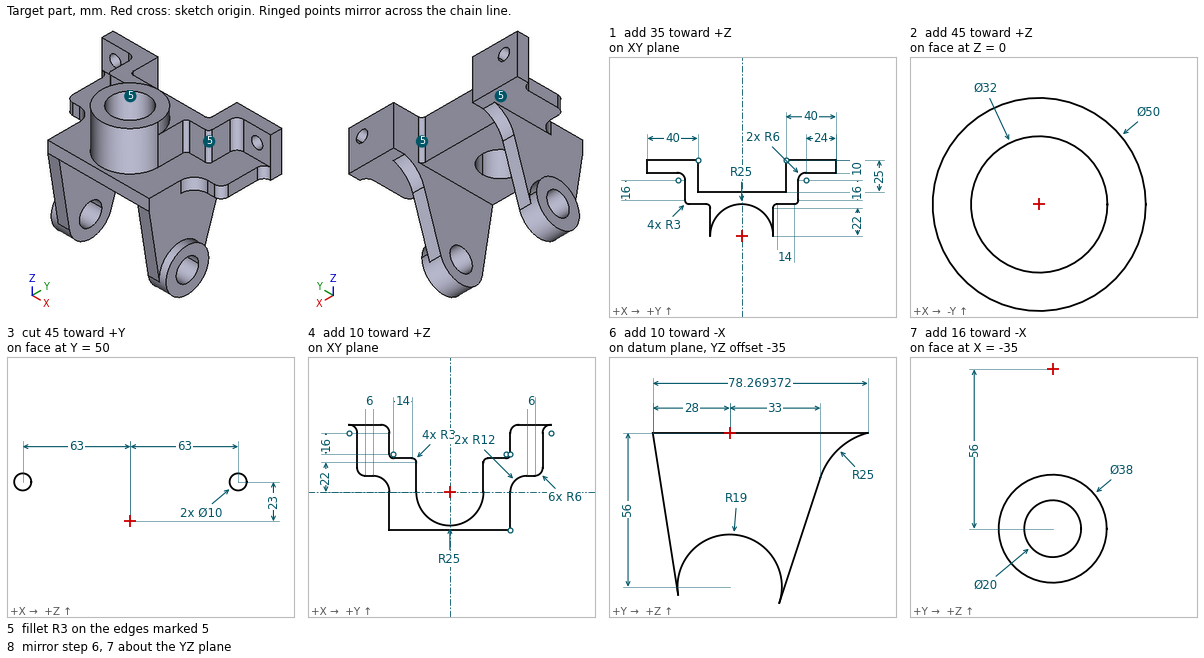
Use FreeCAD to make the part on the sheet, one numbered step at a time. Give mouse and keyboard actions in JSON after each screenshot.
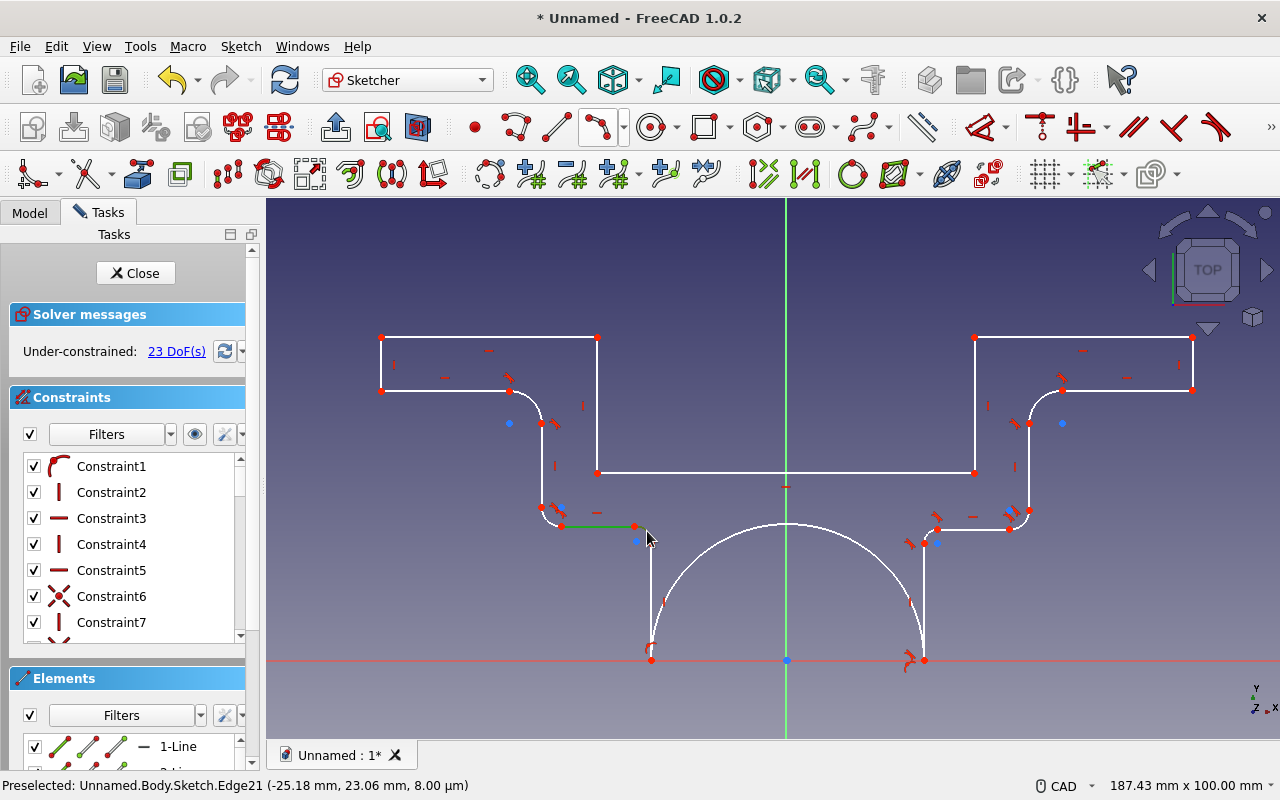
{"action": "left_click", "coordinate": [1216, 128]}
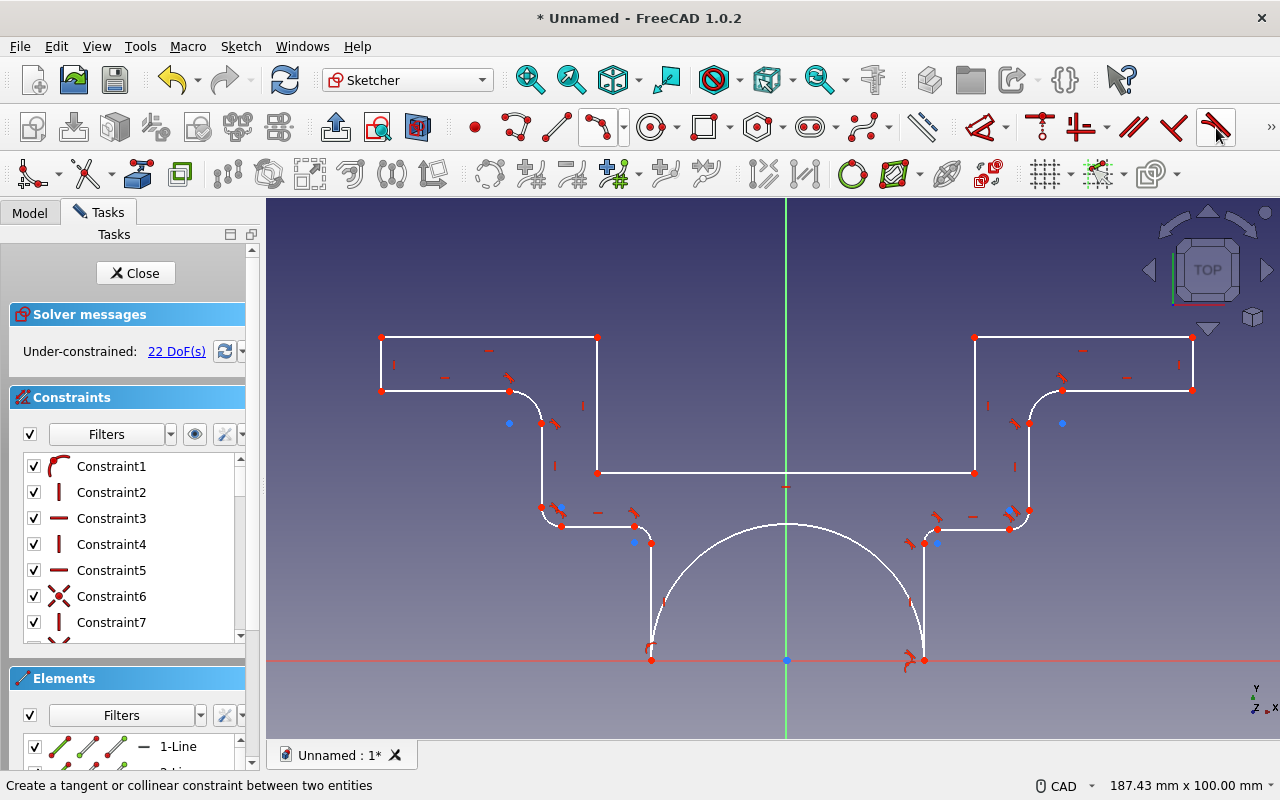
{"action": "left_click", "coordinate": [651, 578]}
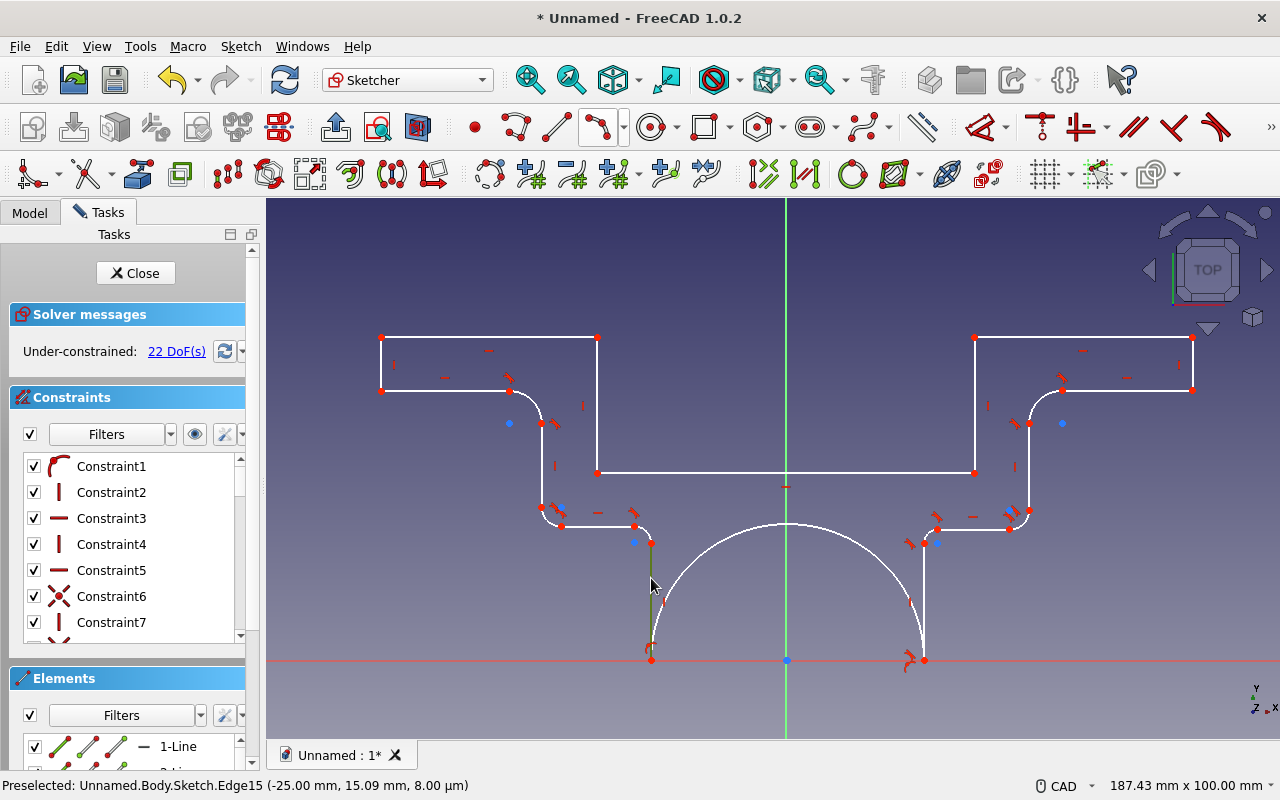
{"action": "left_click", "coordinate": [646, 531]}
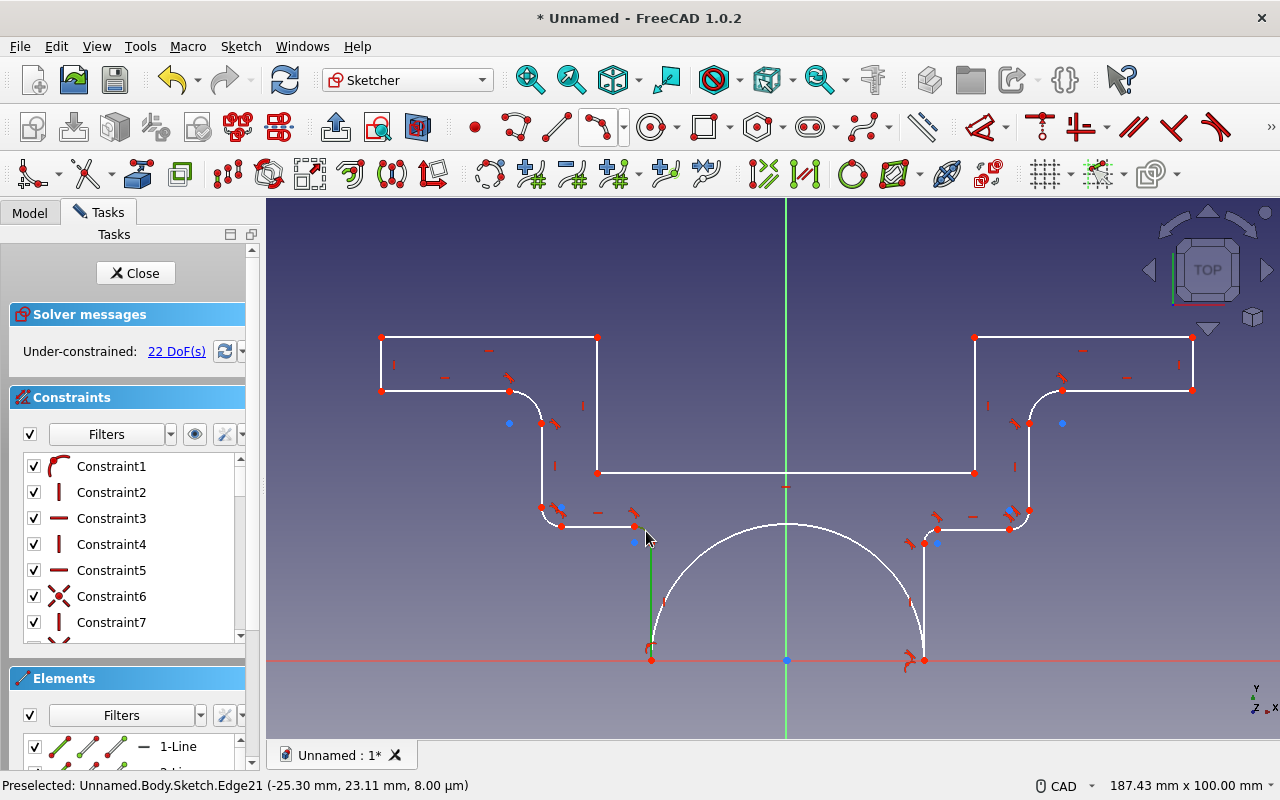
{"action": "left_click", "coordinate": [1216, 128]}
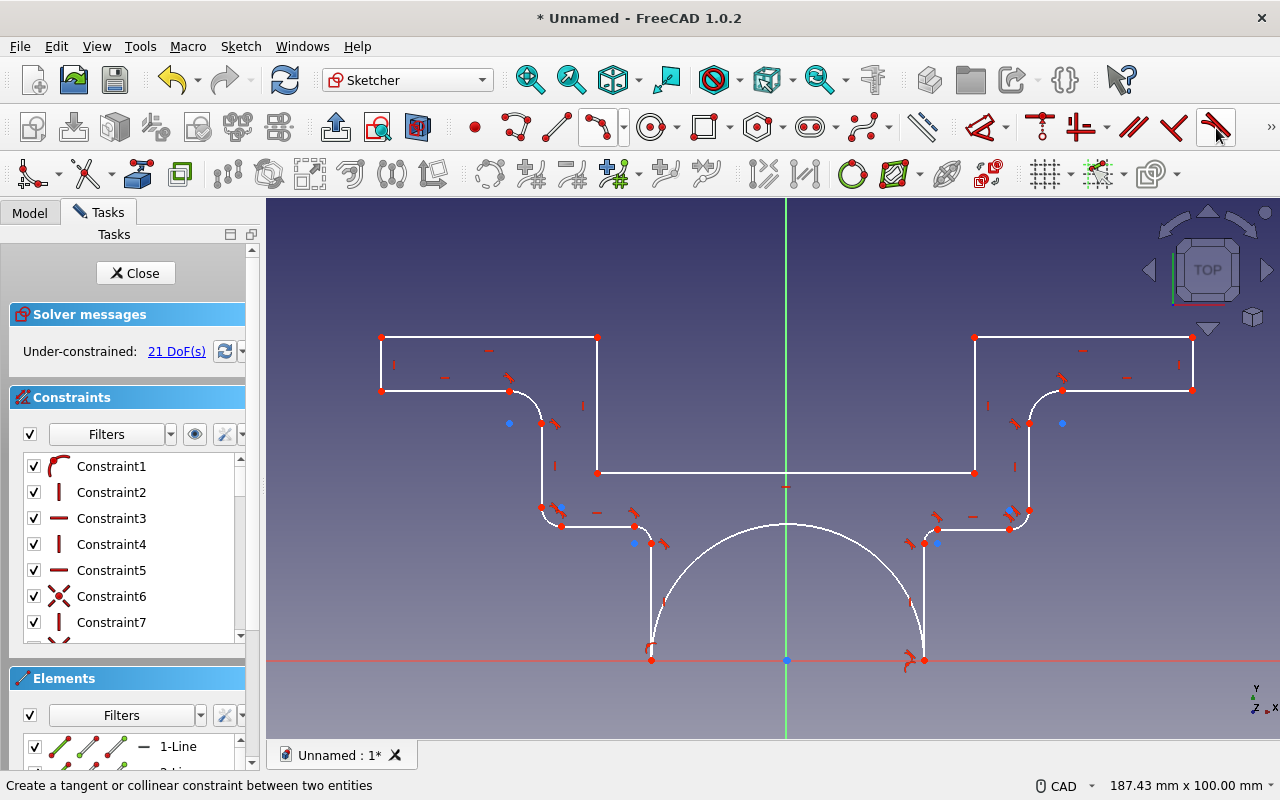
{"action": "scroll", "coordinate": [928, 534], "scroll_direction": "up", "scroll_amount": 2}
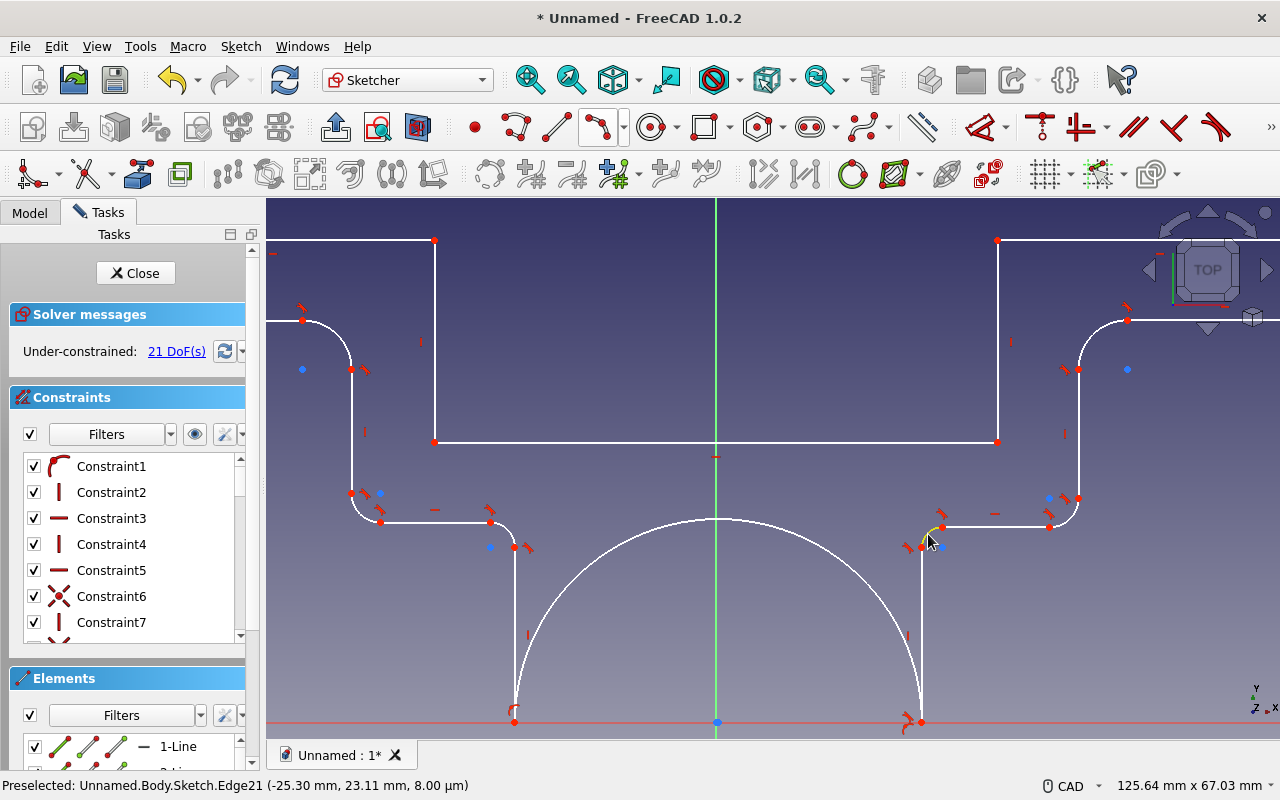
{"action": "left_click", "coordinate": [928, 533]}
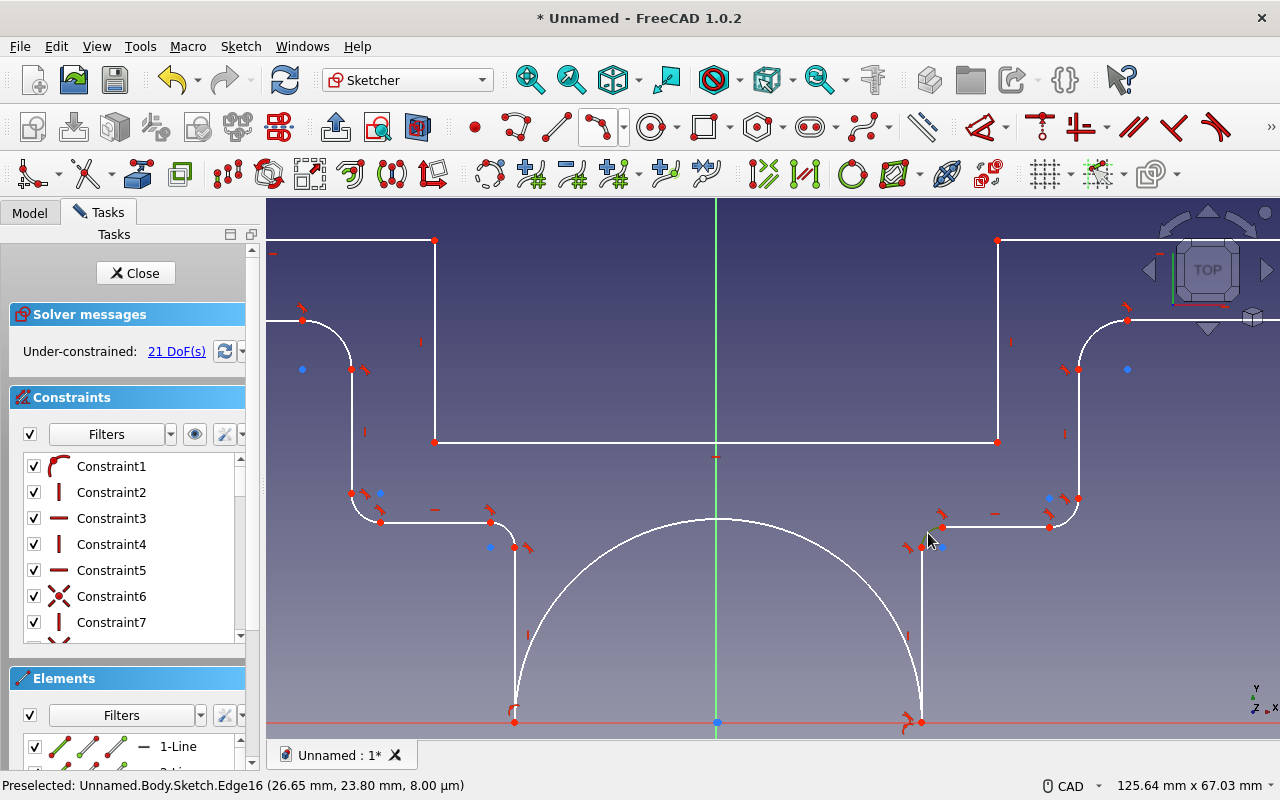
{"action": "left_click", "coordinate": [1063, 524]}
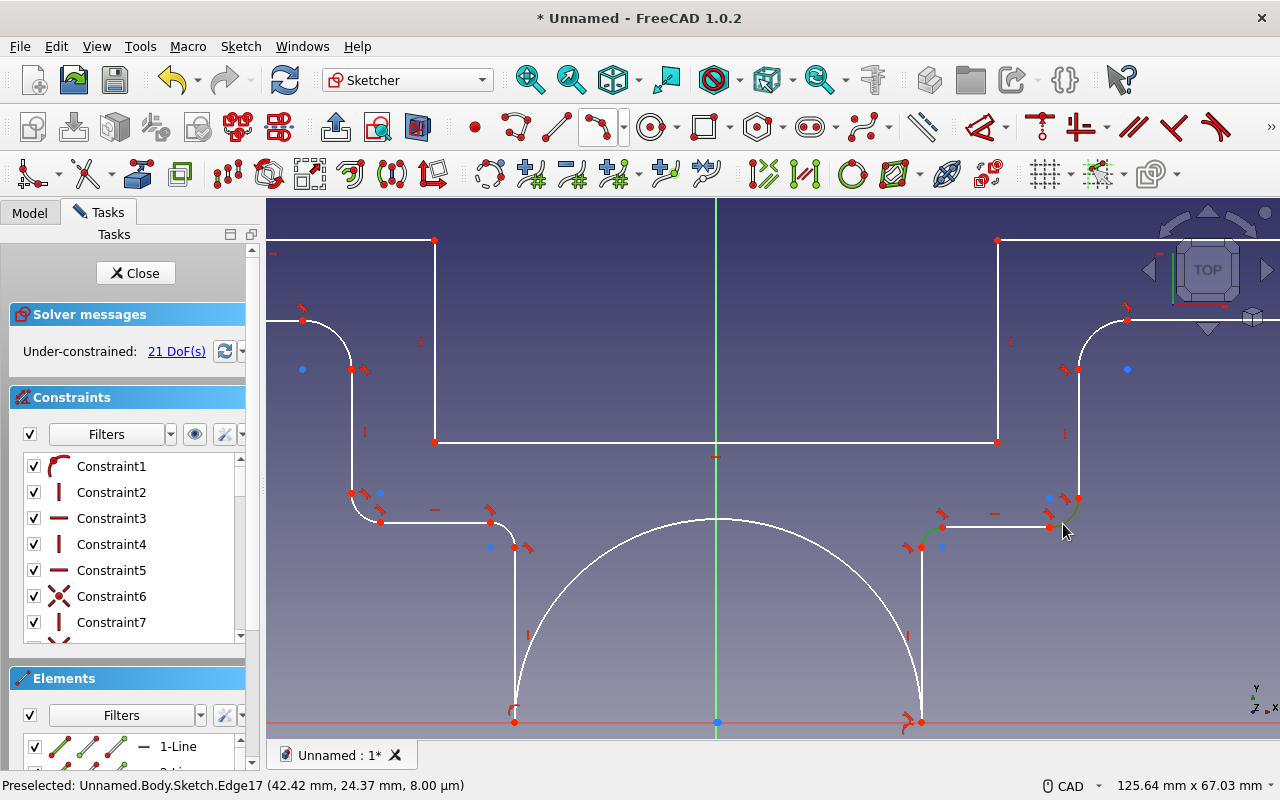
{"action": "left_click", "coordinate": [355, 507]}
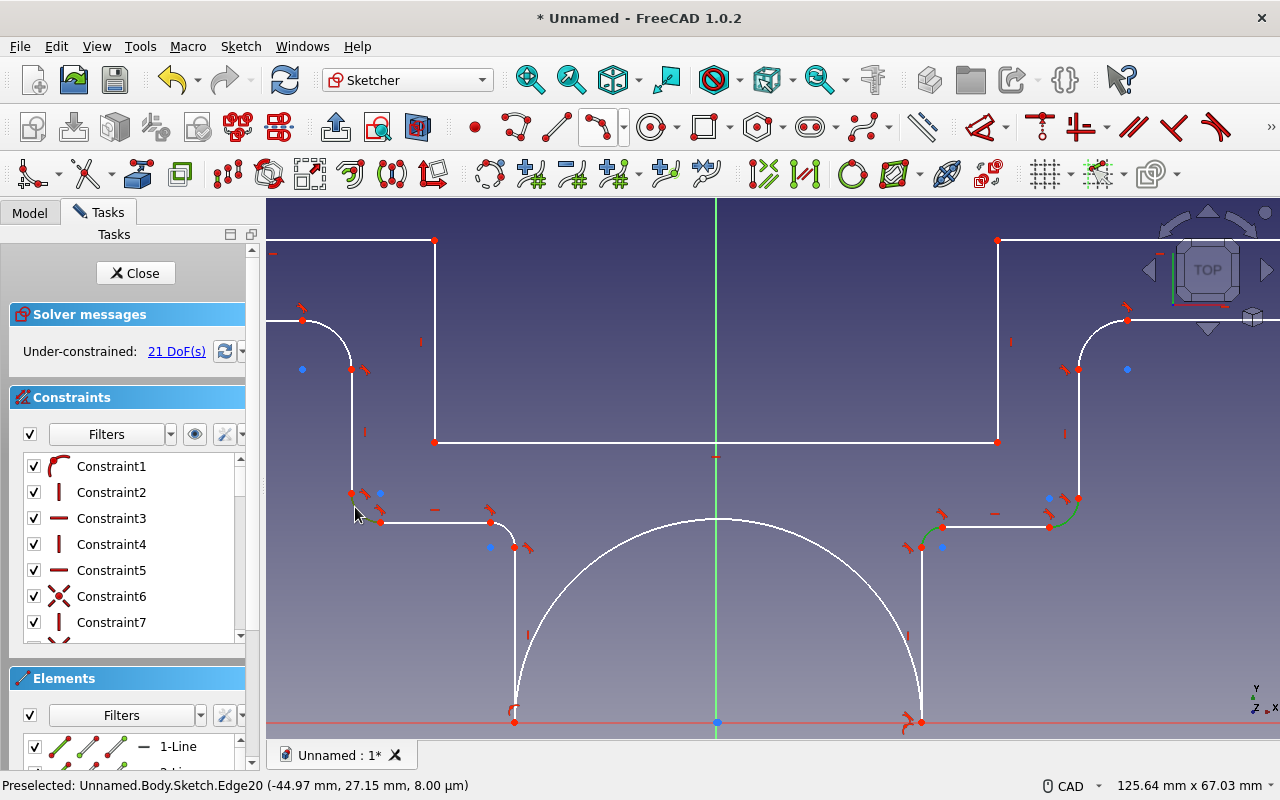
{"action": "left_click", "coordinate": [512, 536]}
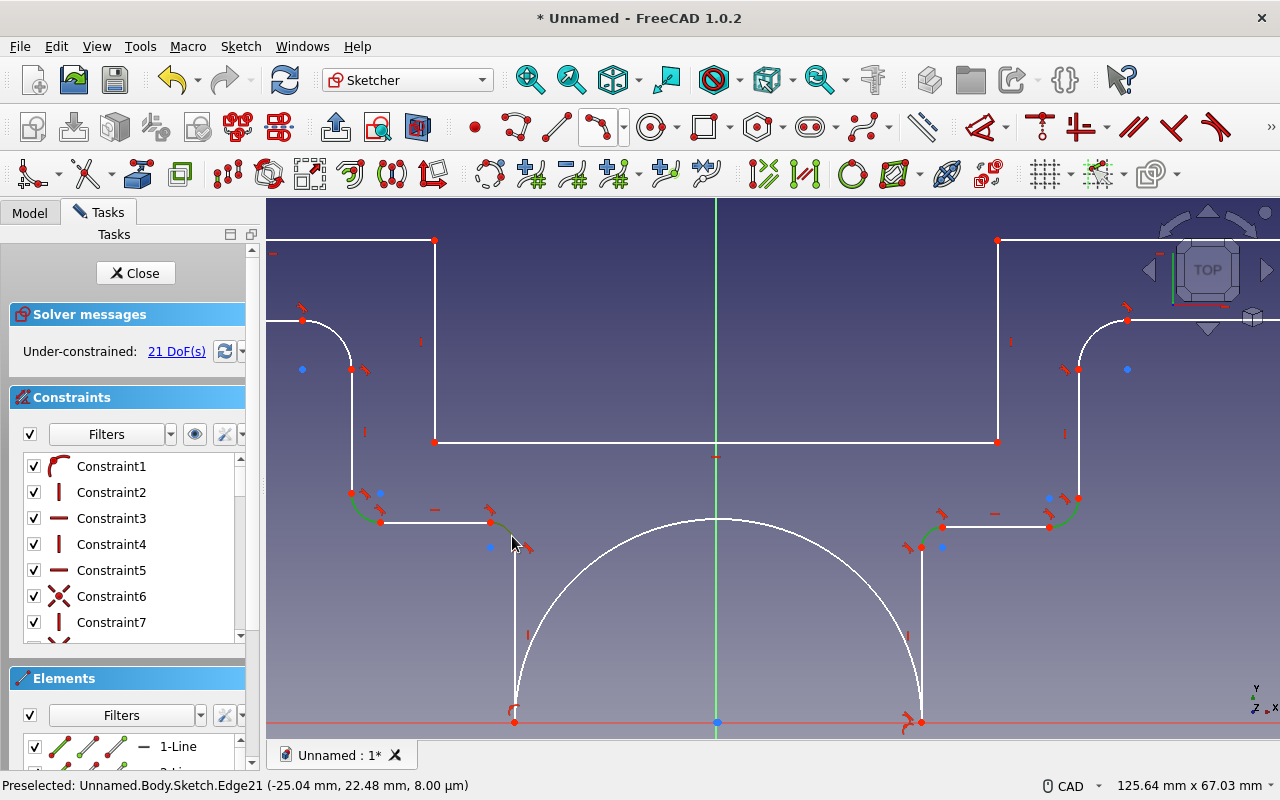
{"action": "key", "text": "e"}